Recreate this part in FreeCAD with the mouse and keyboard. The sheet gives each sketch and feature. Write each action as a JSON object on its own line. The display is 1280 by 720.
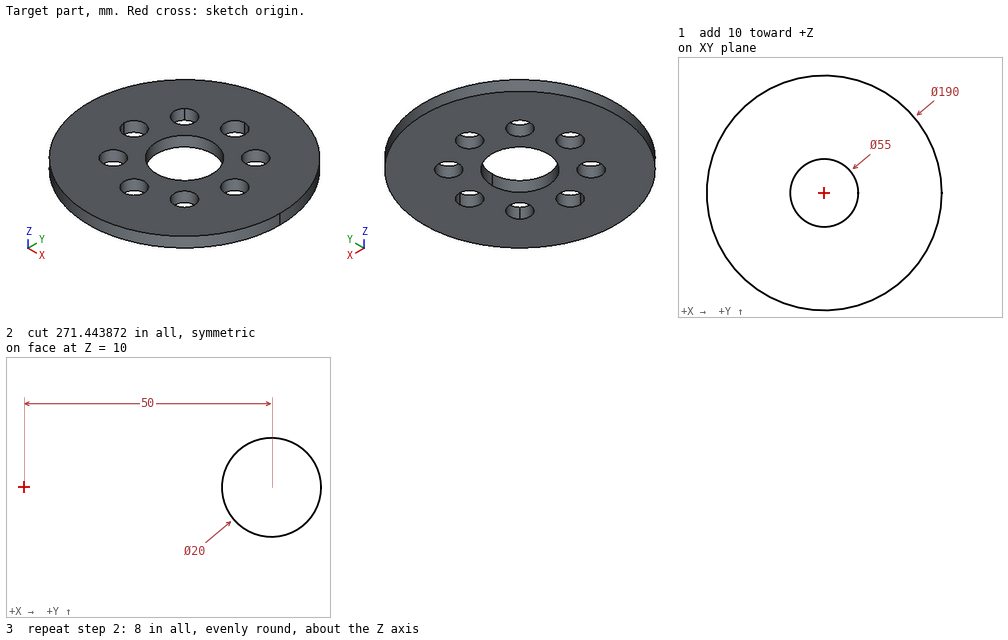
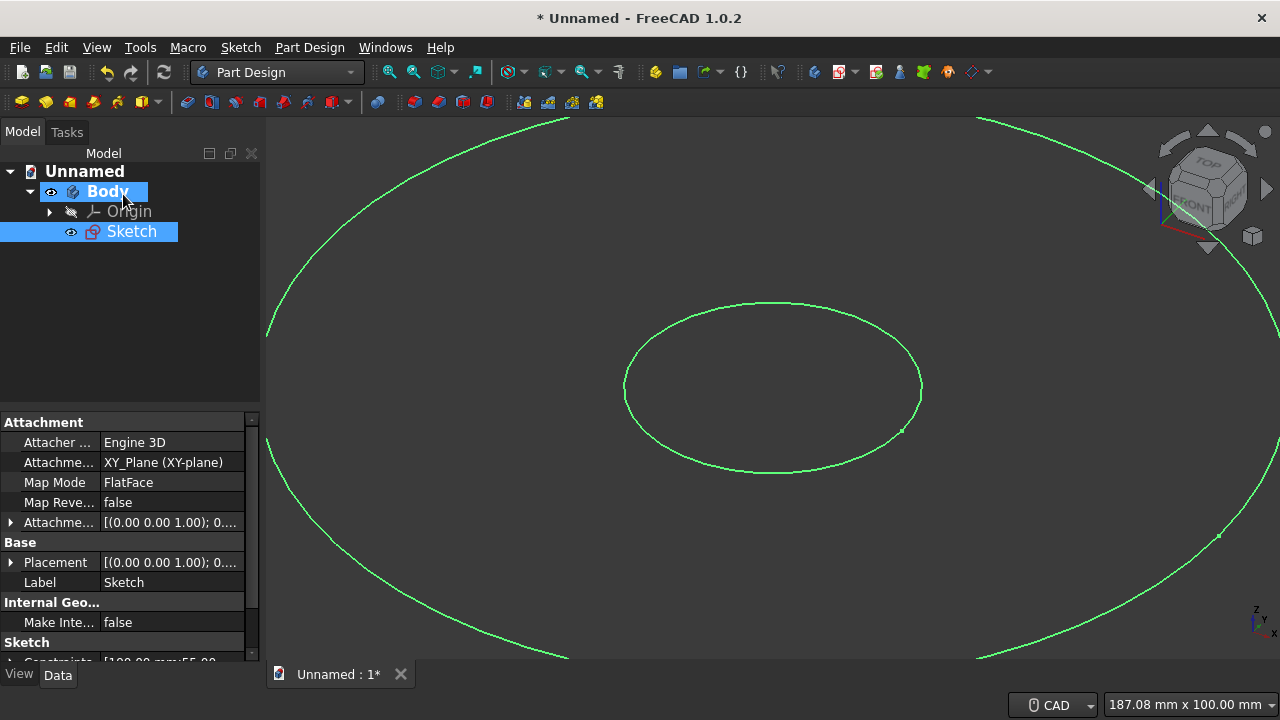
{"action": "left_click", "coordinate": [22, 102]}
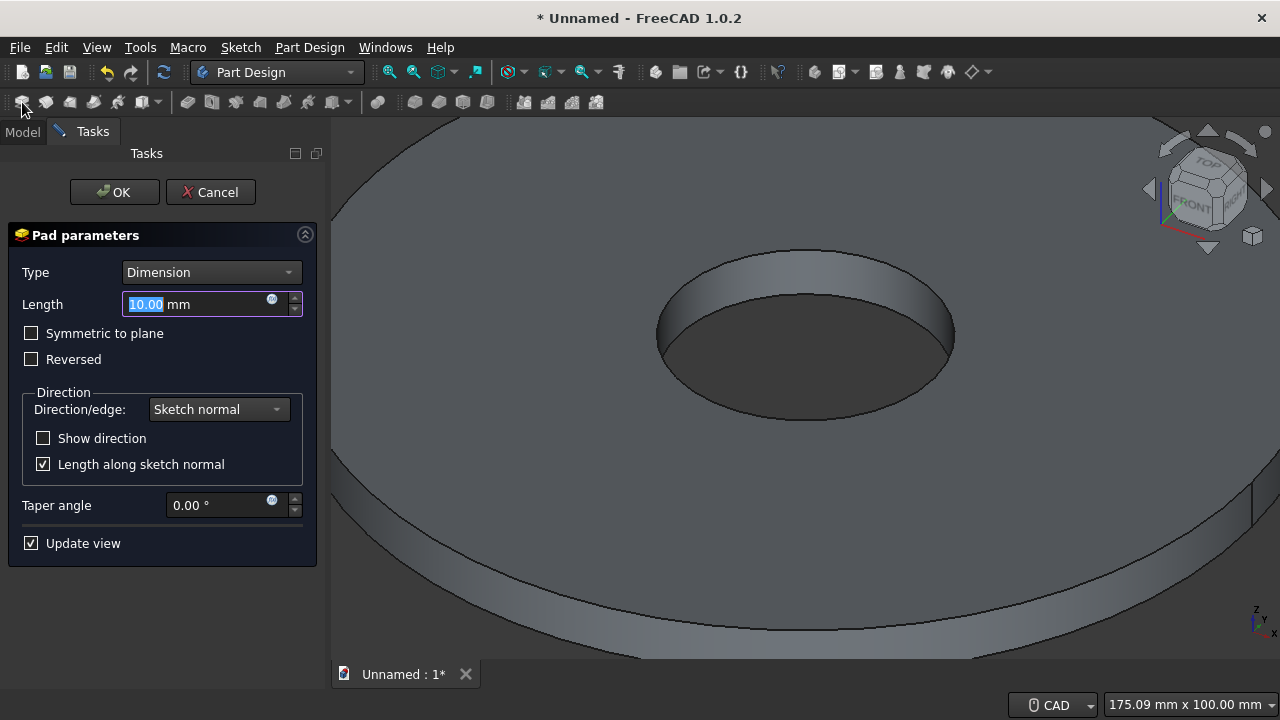
{"action": "type", "text": "10"}
{"action": "key", "text": "Tab"}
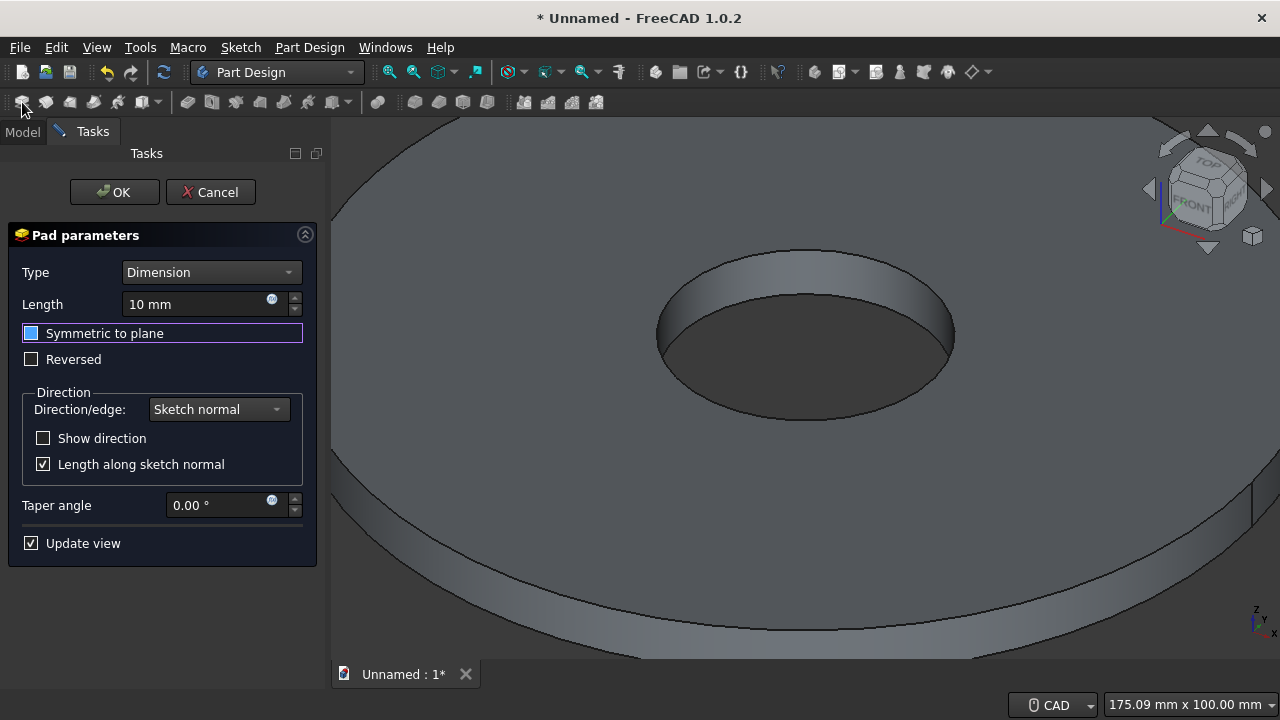
{"action": "left_click", "coordinate": [115, 192]}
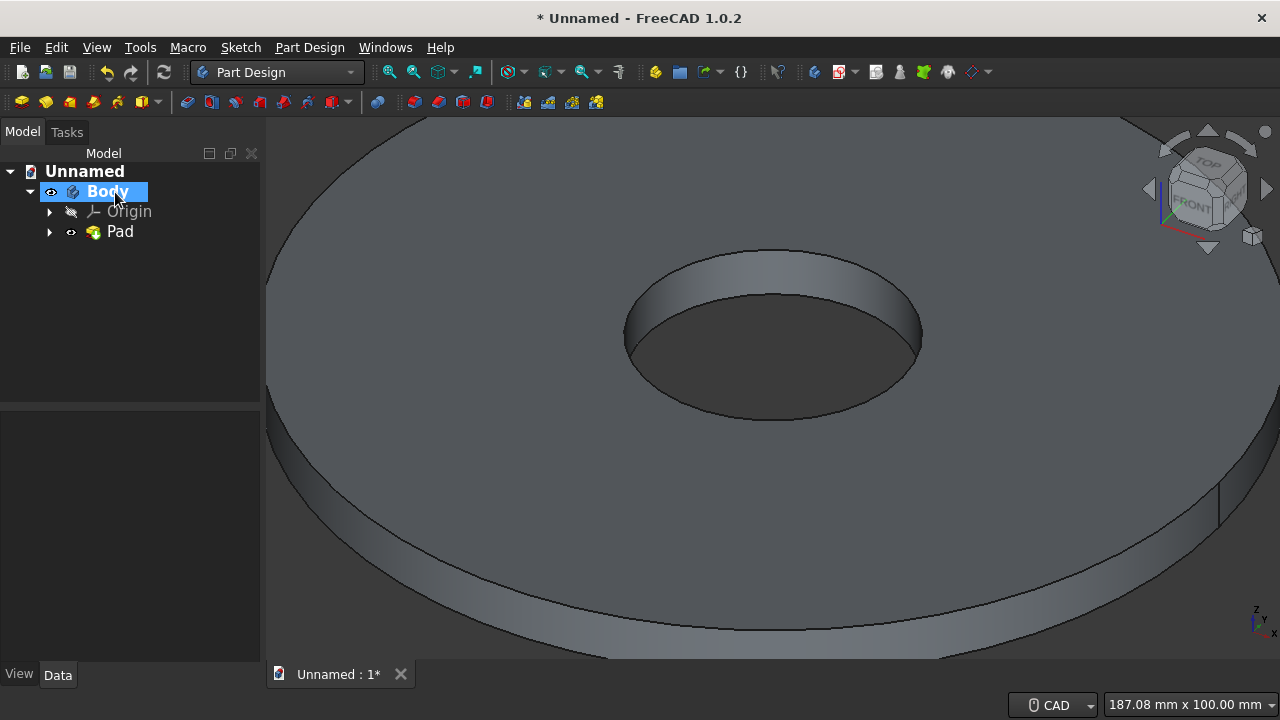
{"action": "left_click", "coordinate": [390, 72]}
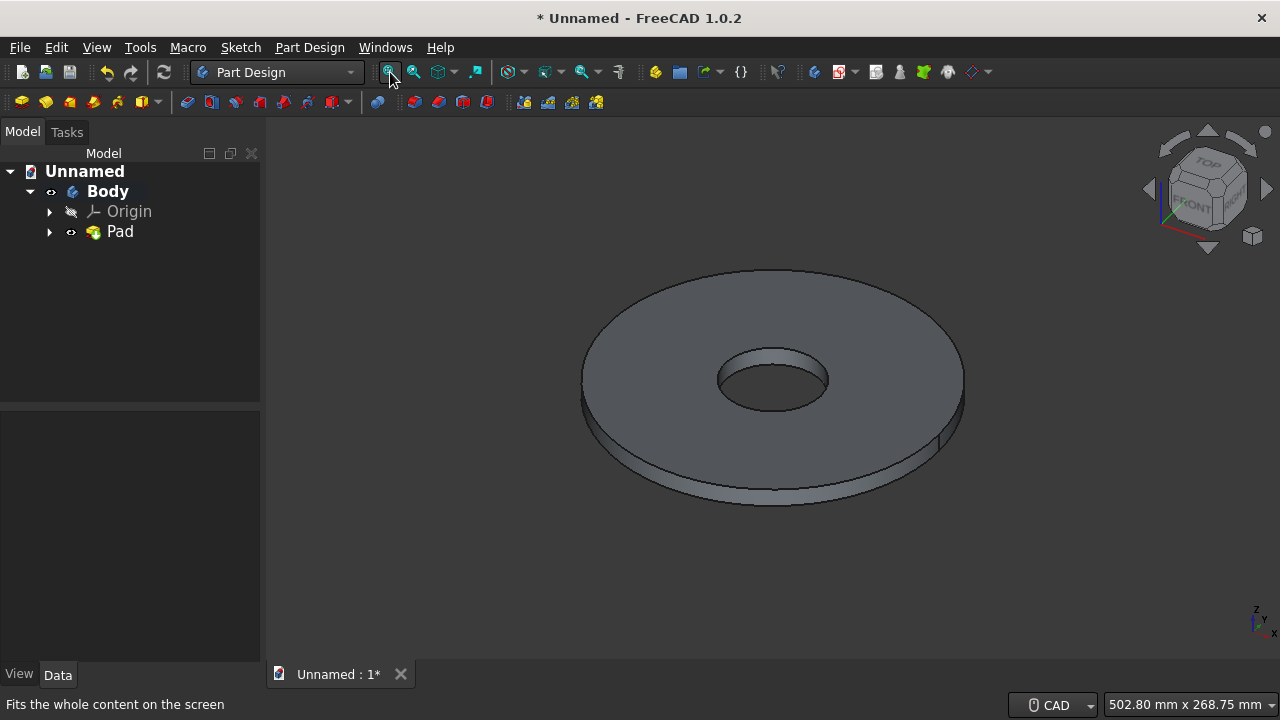
{"action": "left_click", "coordinate": [705, 320]}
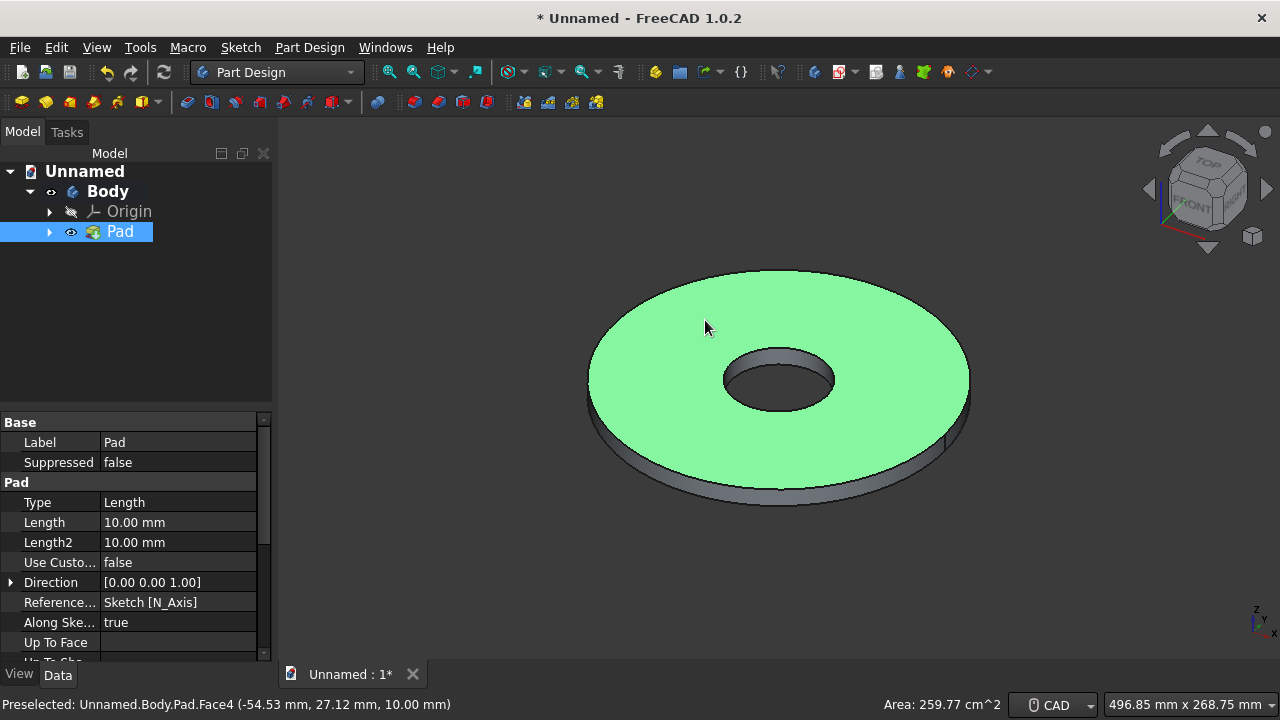
{"action": "left_click", "coordinate": [840, 72]}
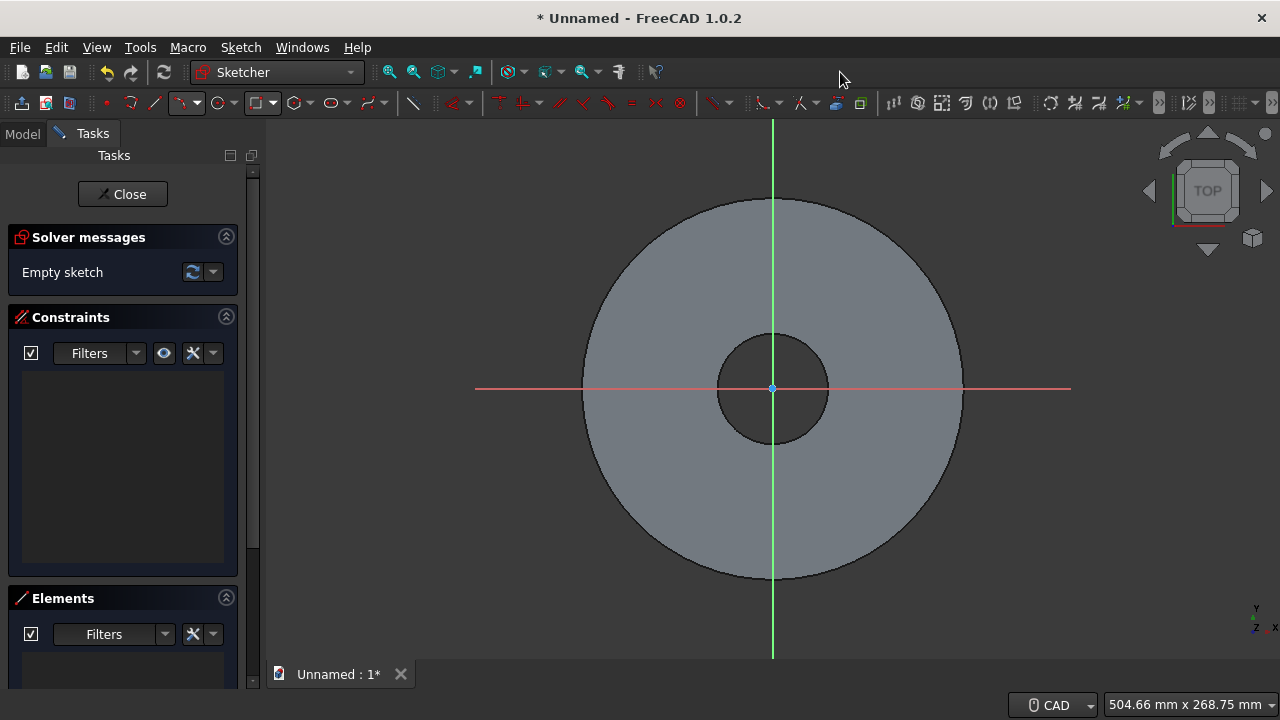
{"action": "scroll", "coordinate": [894, 389], "scroll_direction": "up", "scroll_amount": 11}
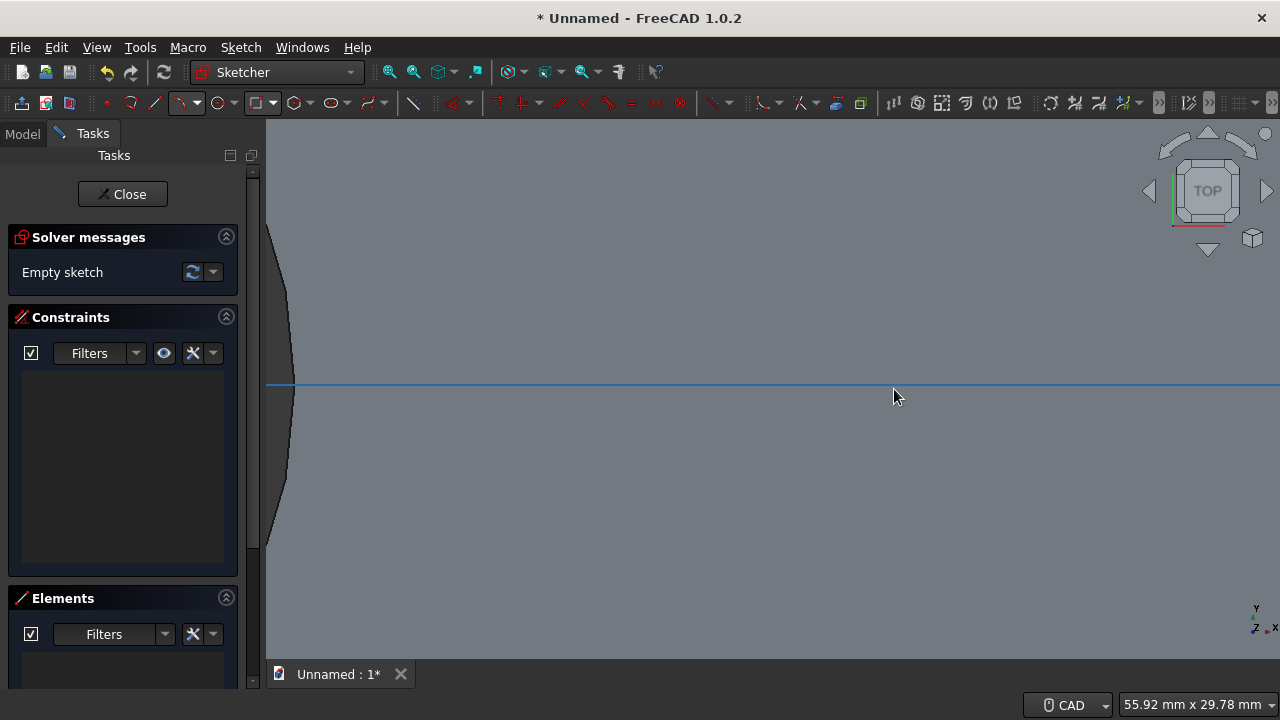
{"action": "left_click", "coordinate": [218, 104]}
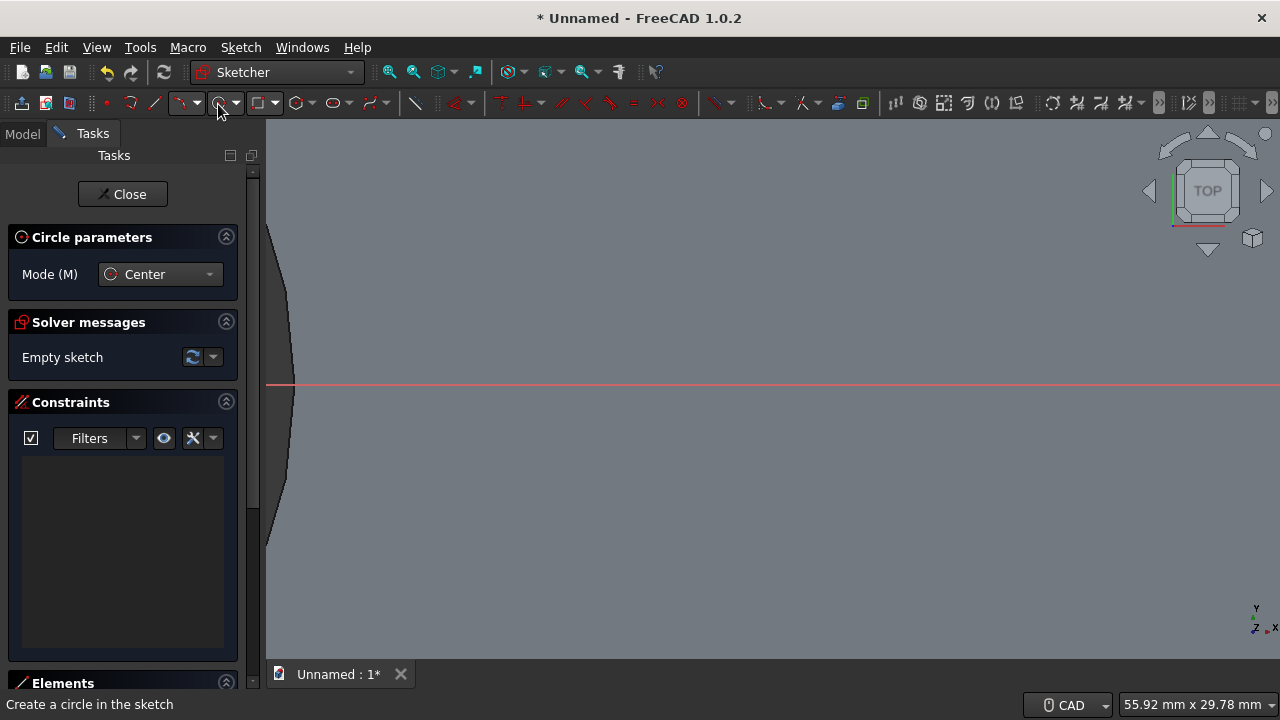
{"action": "left_click", "coordinate": [703, 385]}
{"action": "mouse_move", "coordinate": [831, 257]}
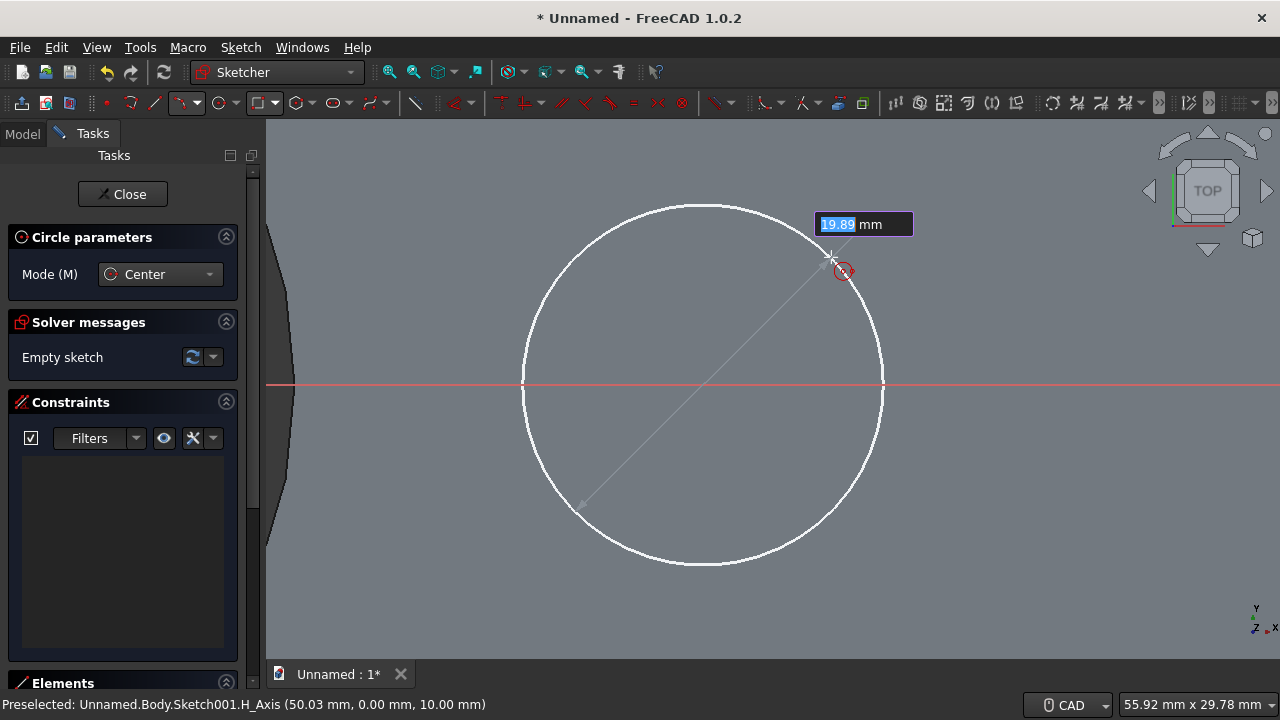
{"action": "type", "text": "20"}
{"action": "key", "text": "Return"}
{"action": "key", "text": "Escape"}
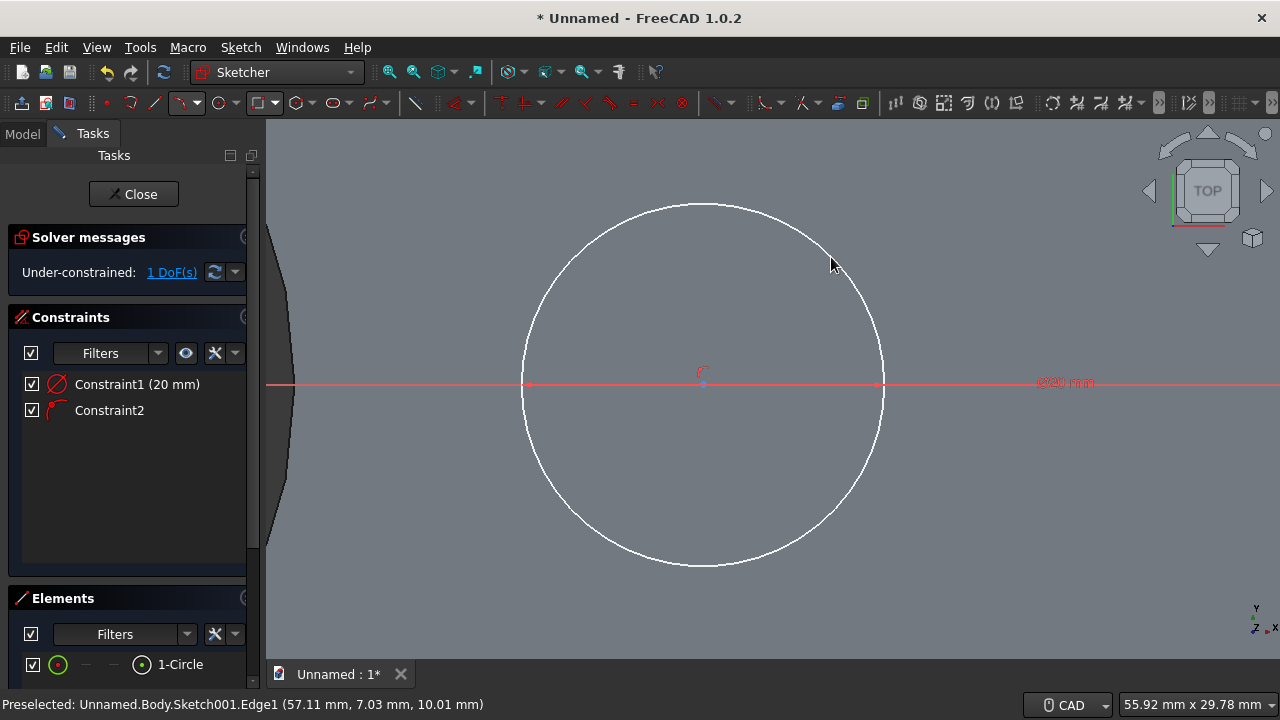
{"action": "left_click", "coordinate": [454, 104]}